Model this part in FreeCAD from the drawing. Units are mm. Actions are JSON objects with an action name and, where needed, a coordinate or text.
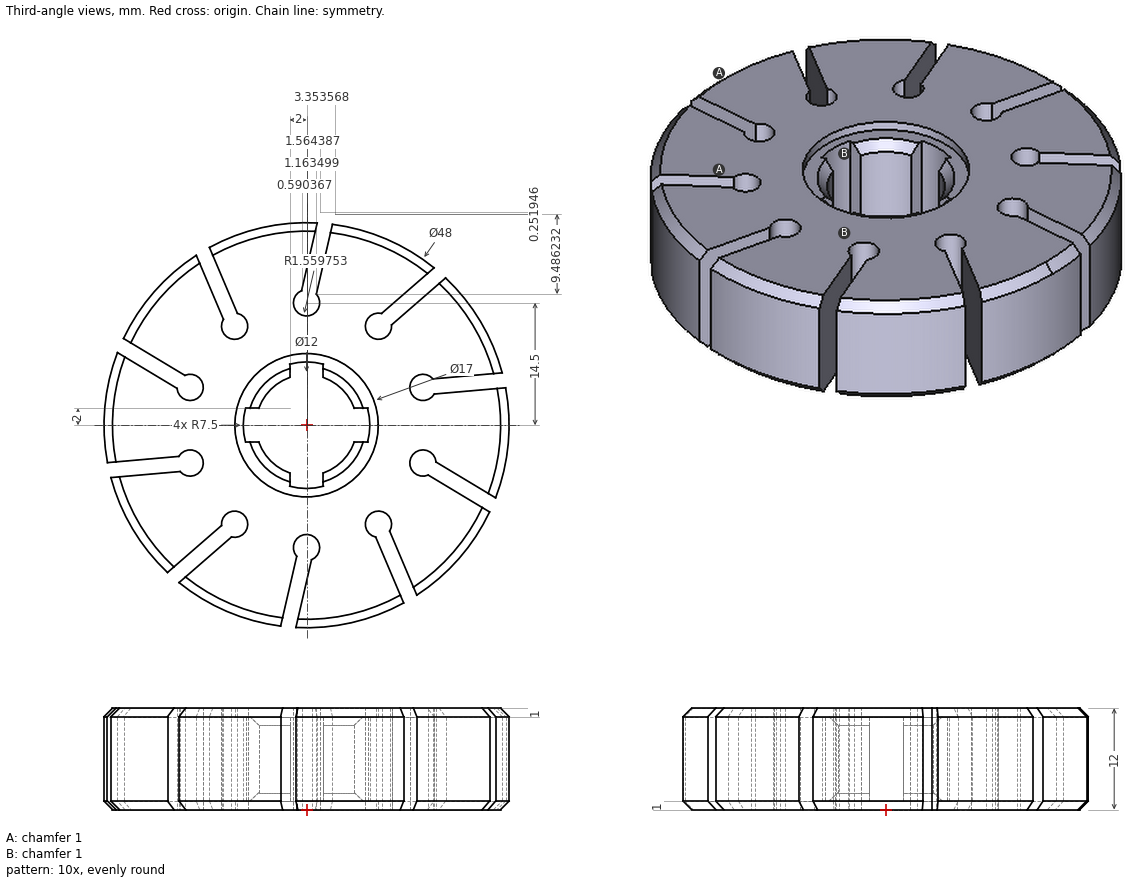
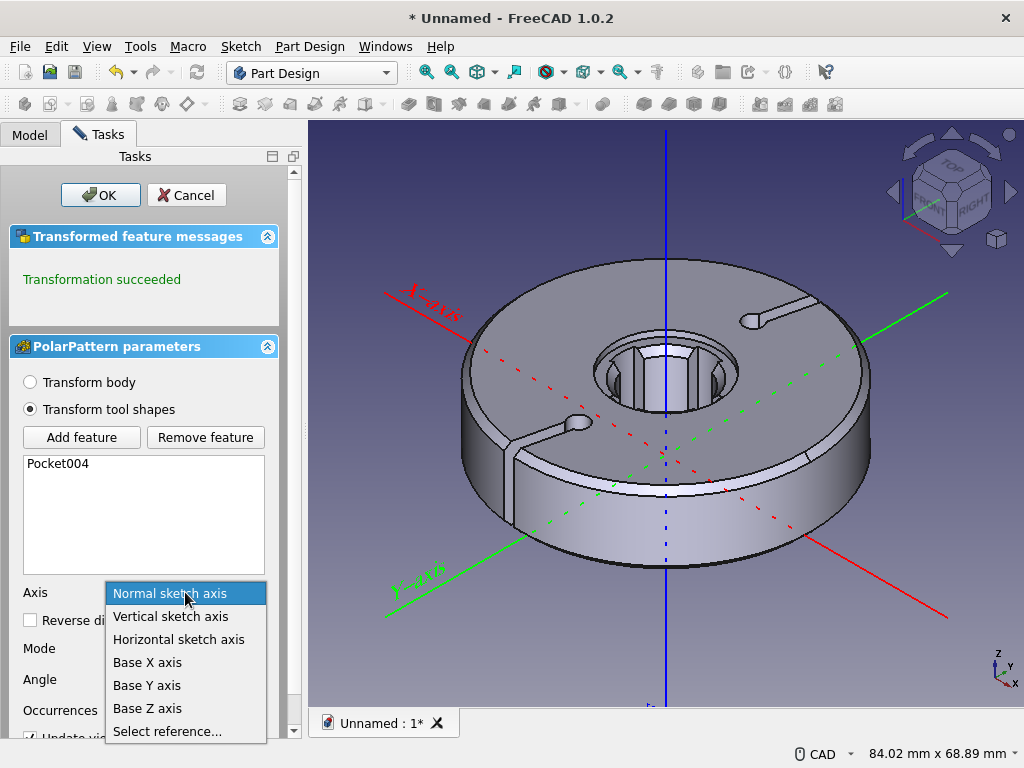
{"action": "left_click", "coordinate": [184, 708]}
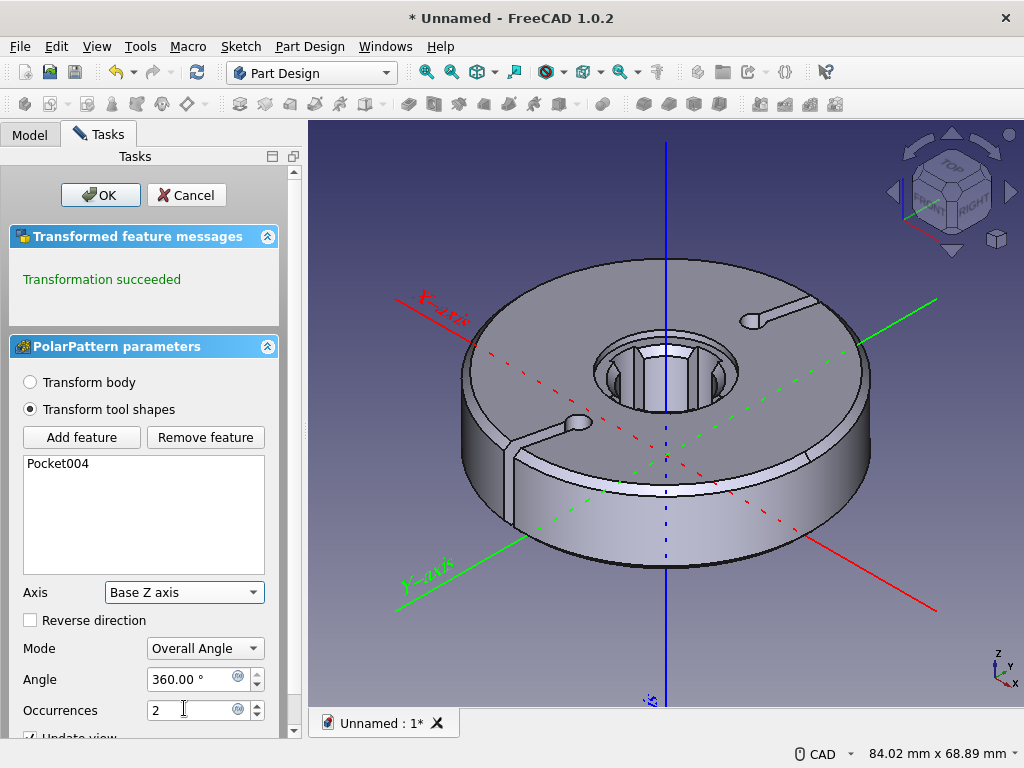
{"action": "triple_click", "coordinate": [199, 710]}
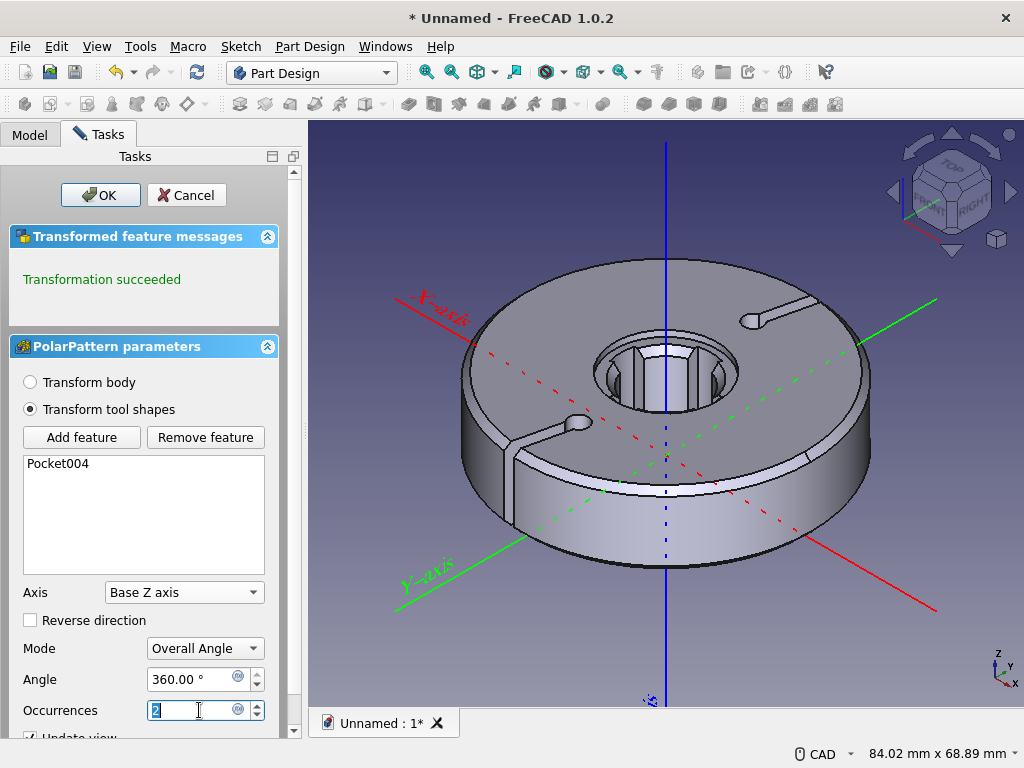
{"action": "type", "text": "10"}
{"action": "key", "text": "Tab"}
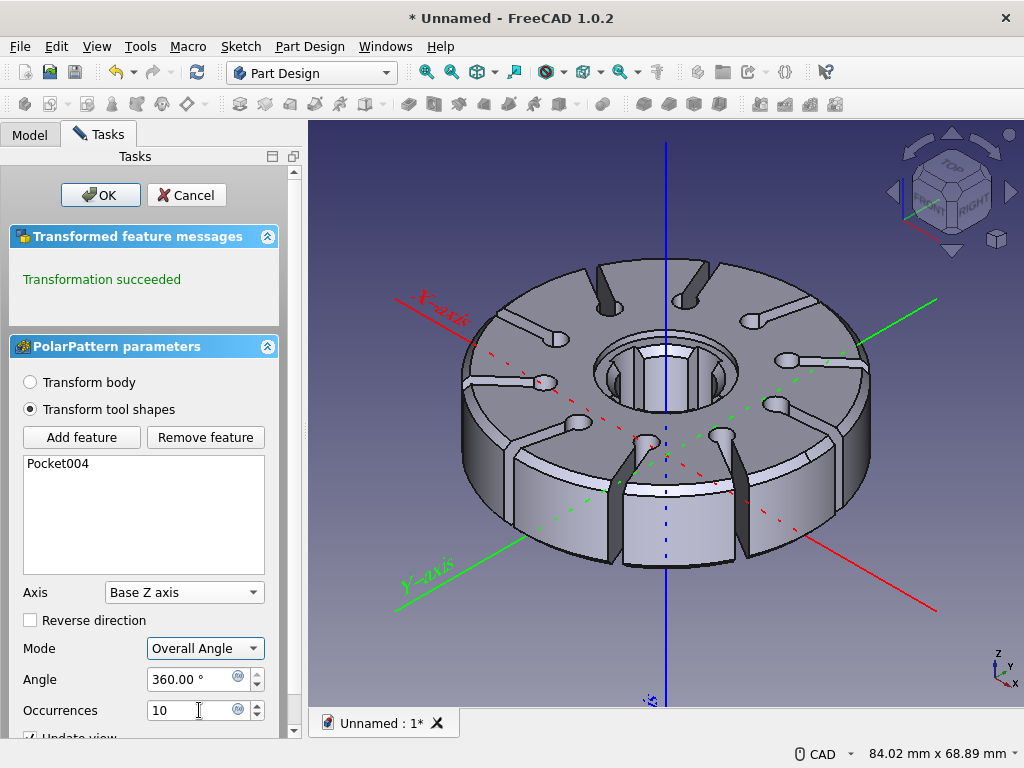
{"action": "left_click", "coordinate": [101, 195]}